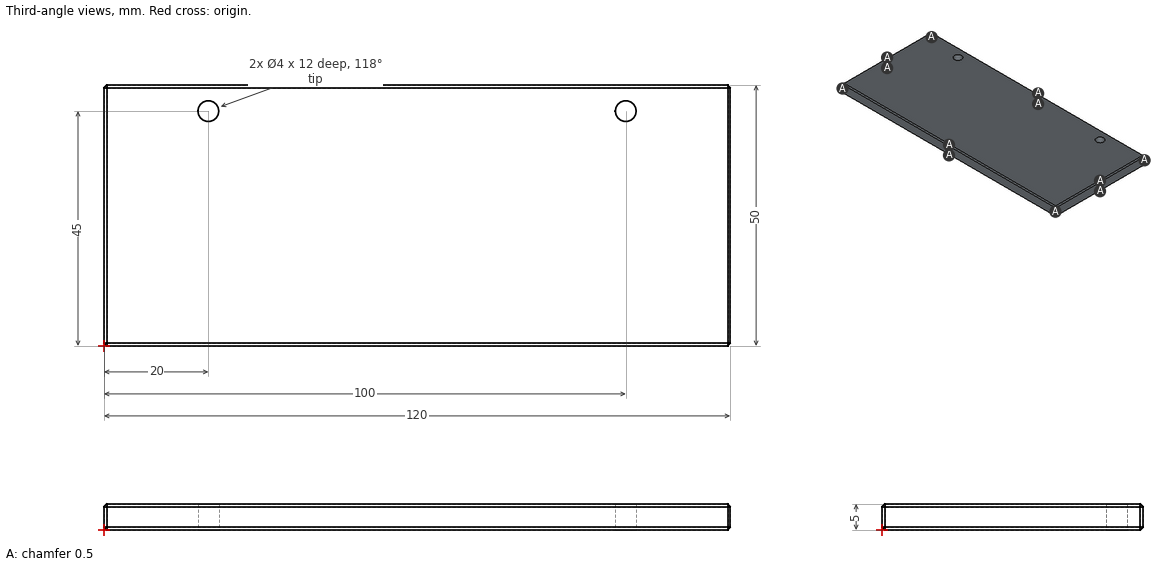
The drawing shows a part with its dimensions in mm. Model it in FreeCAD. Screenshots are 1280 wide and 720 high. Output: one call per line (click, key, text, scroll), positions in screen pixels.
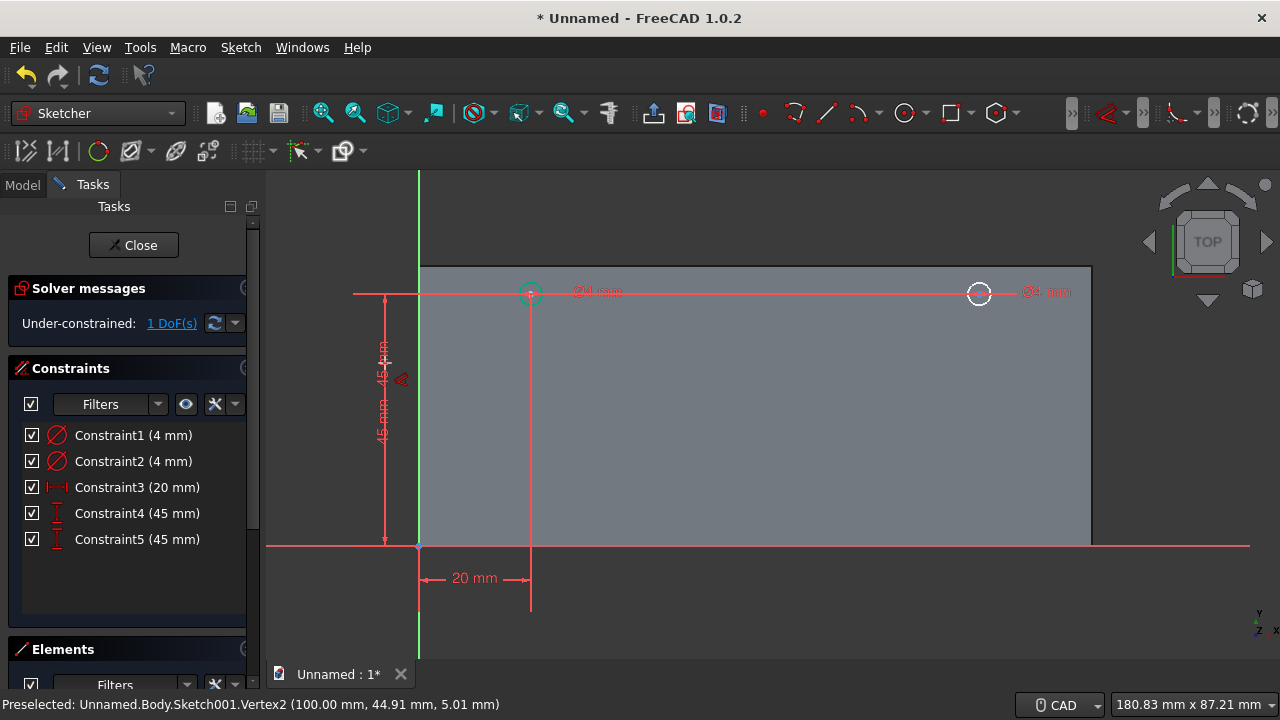
click(979, 294)
click(699, 580)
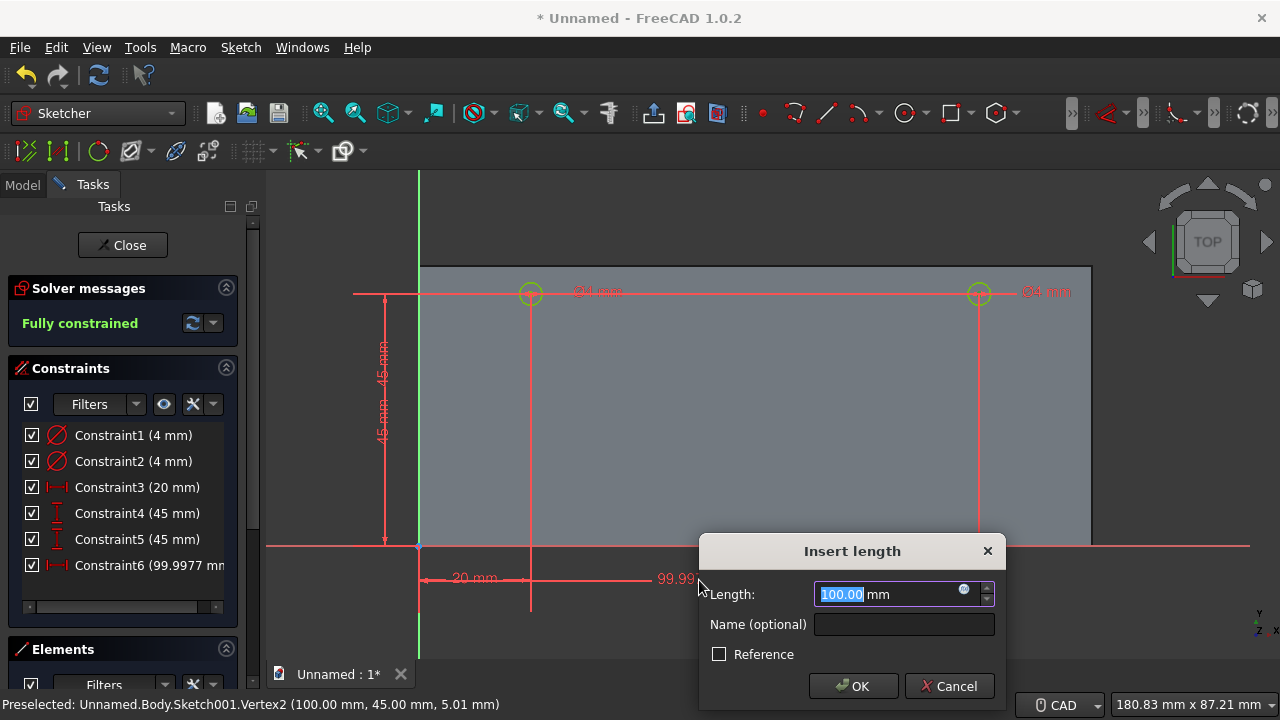
text(100)
key(Return)
key(Escape)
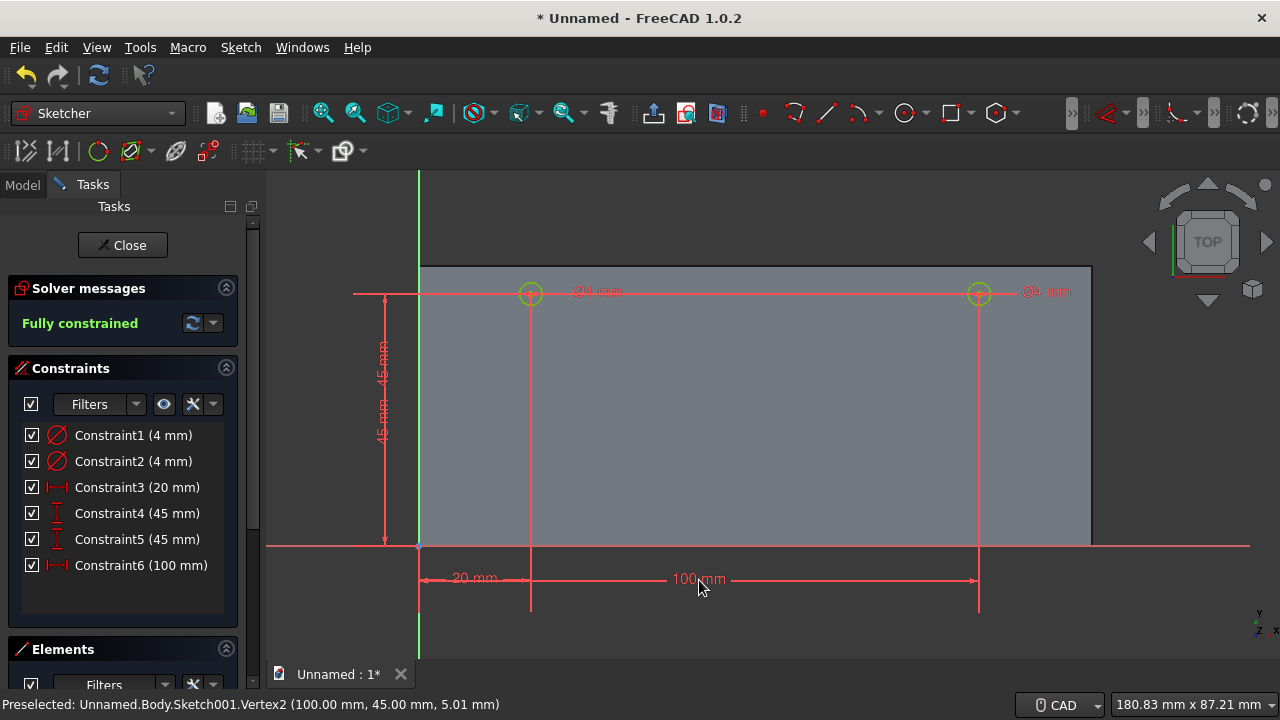
click(123, 245)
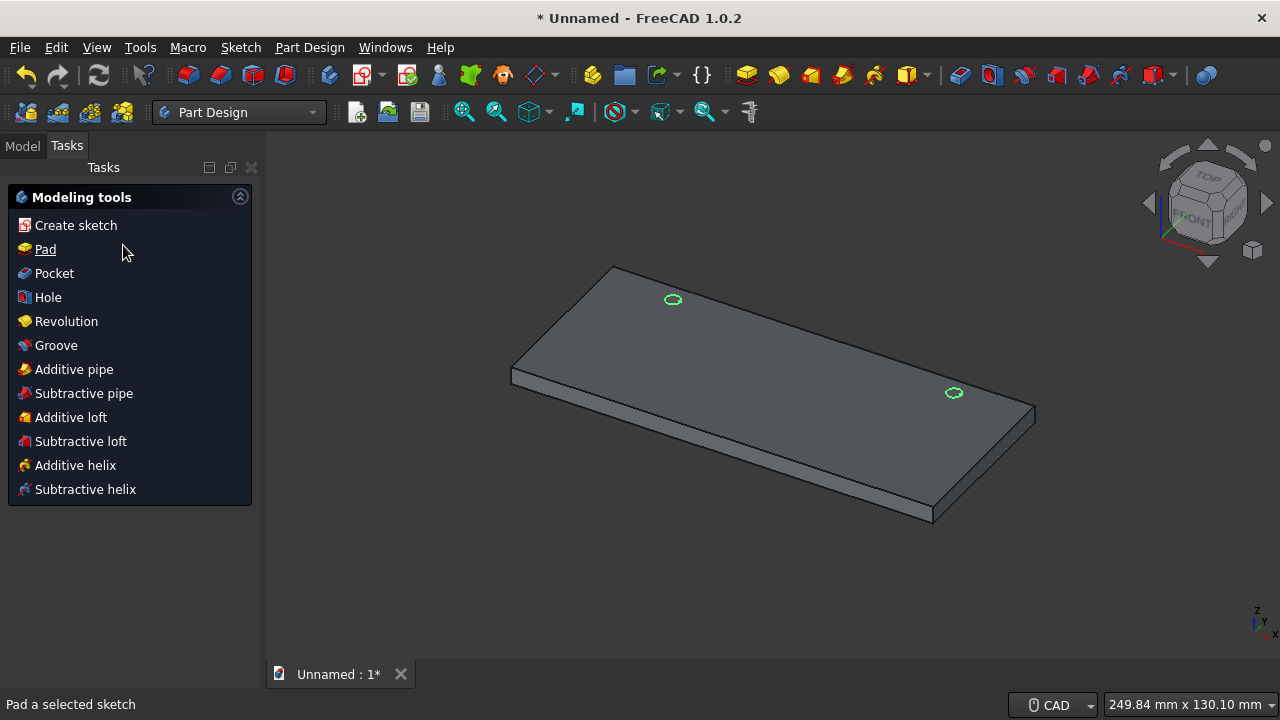
click(994, 76)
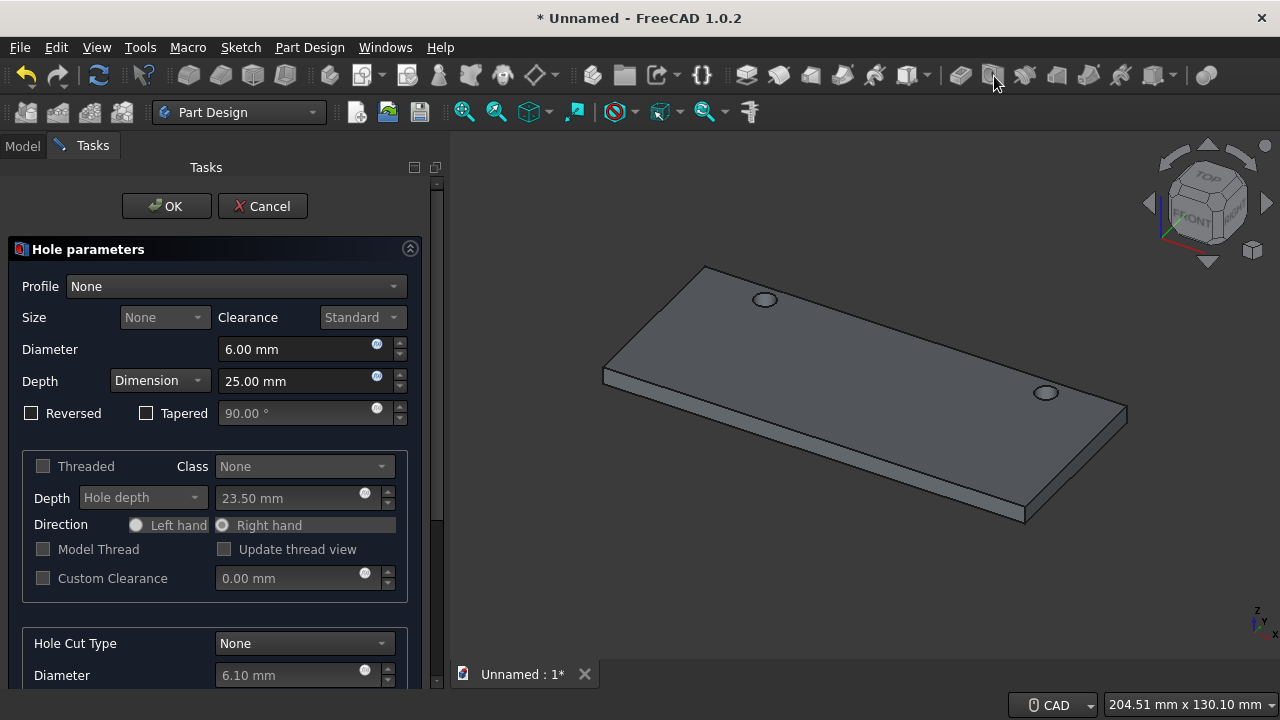
triple_click(305, 349)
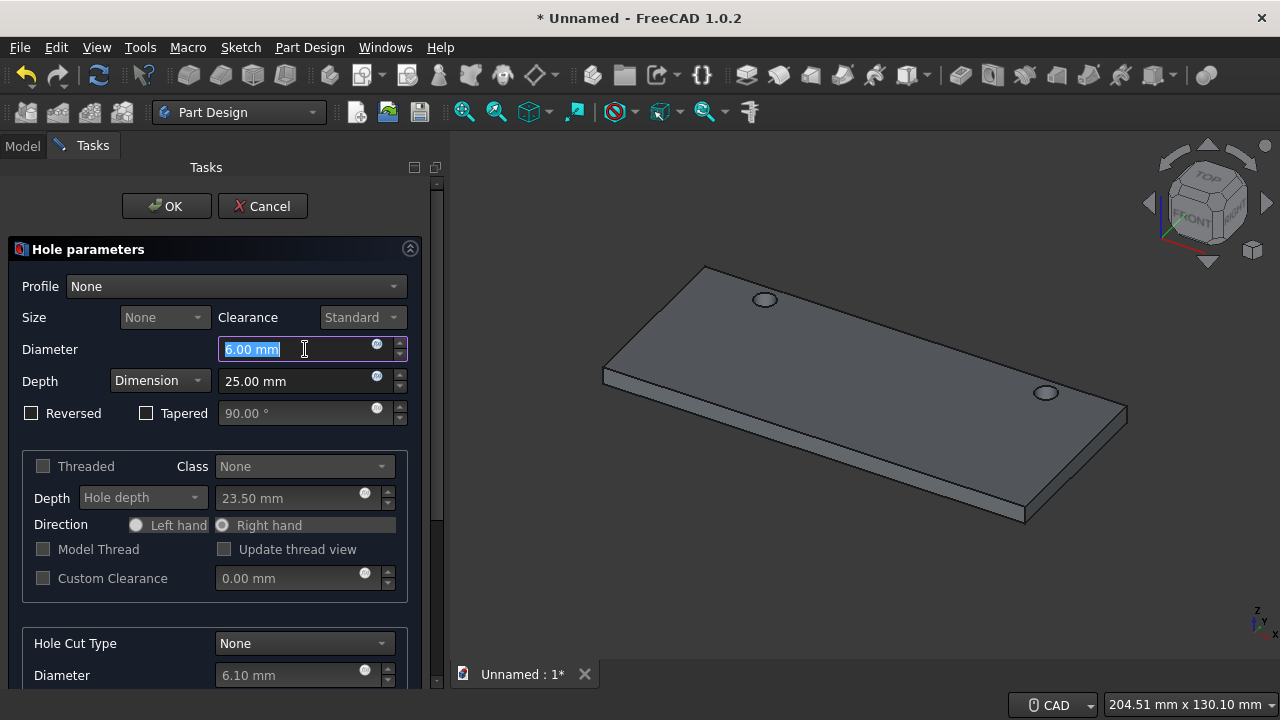
text(4)
key(Tab)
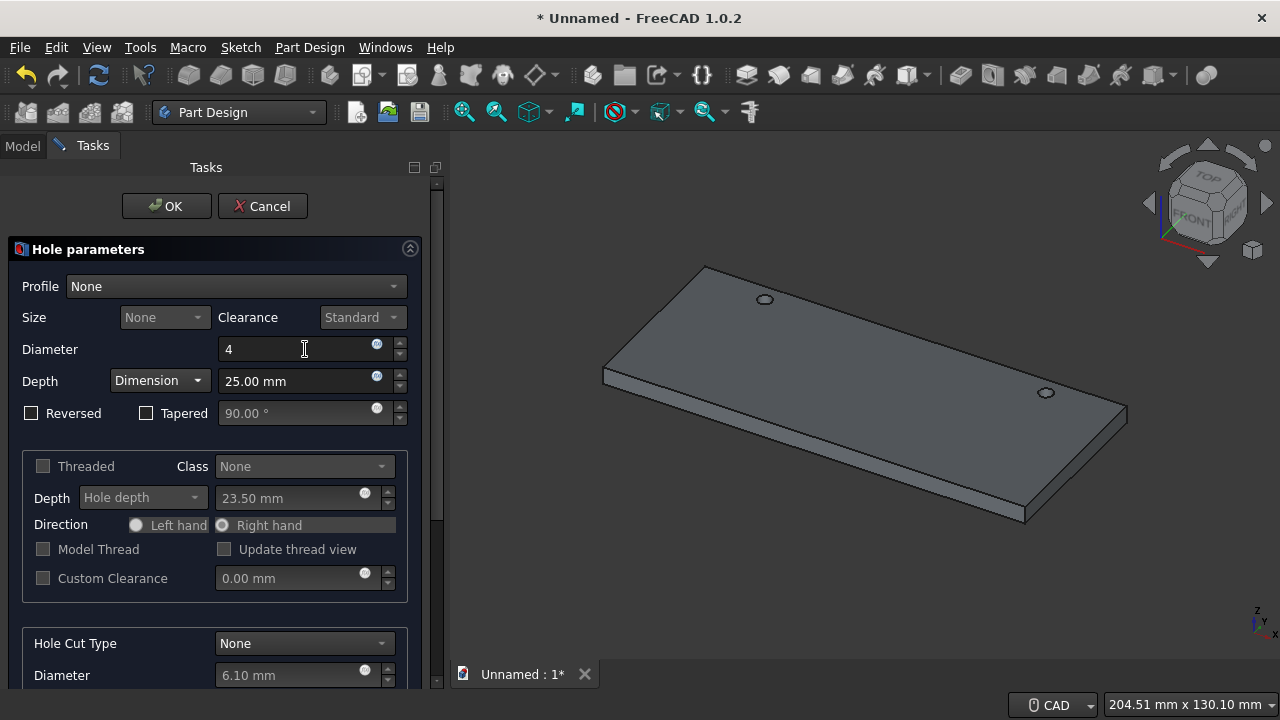
triple_click(305, 381)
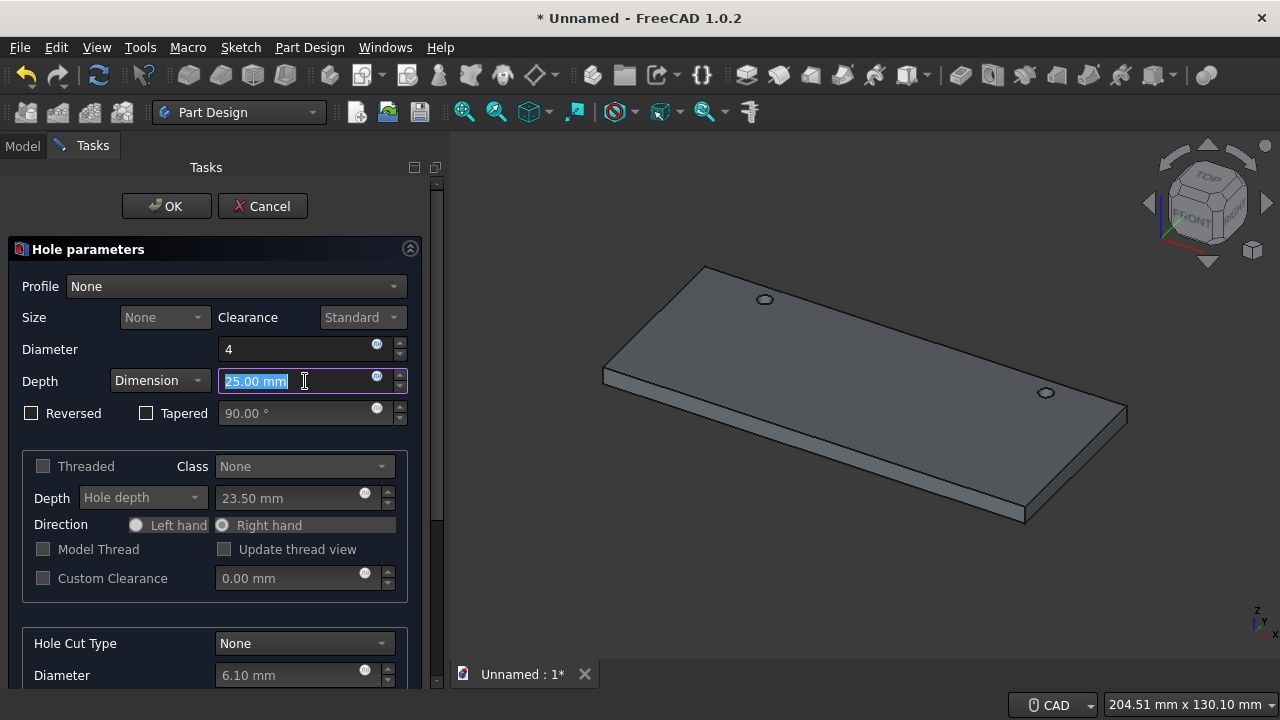
text(12)
key(Tab)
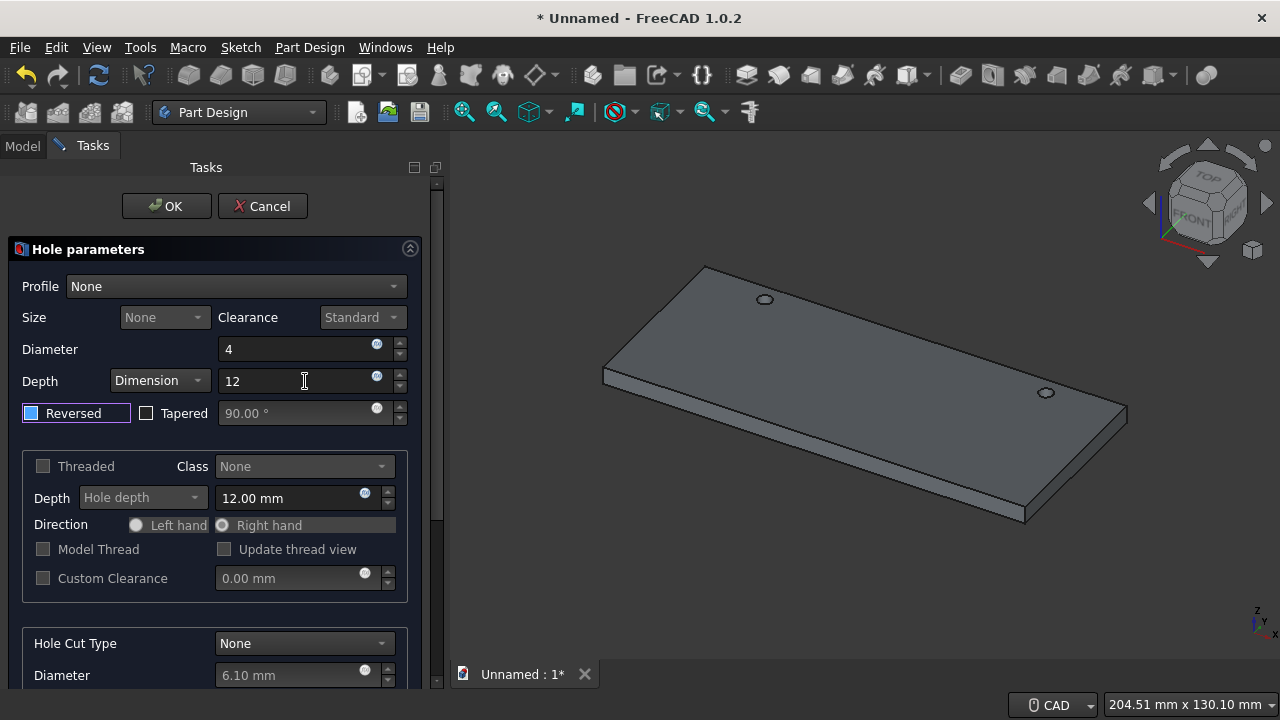
click(167, 206)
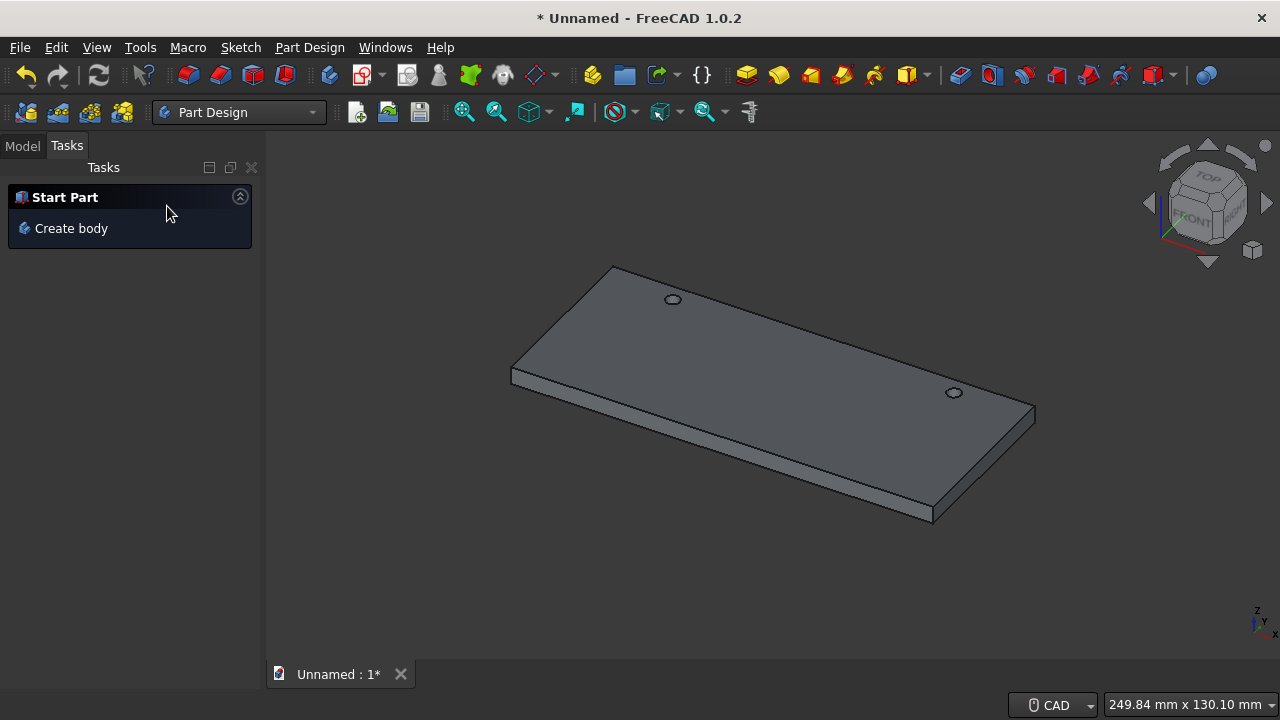
click(984, 456)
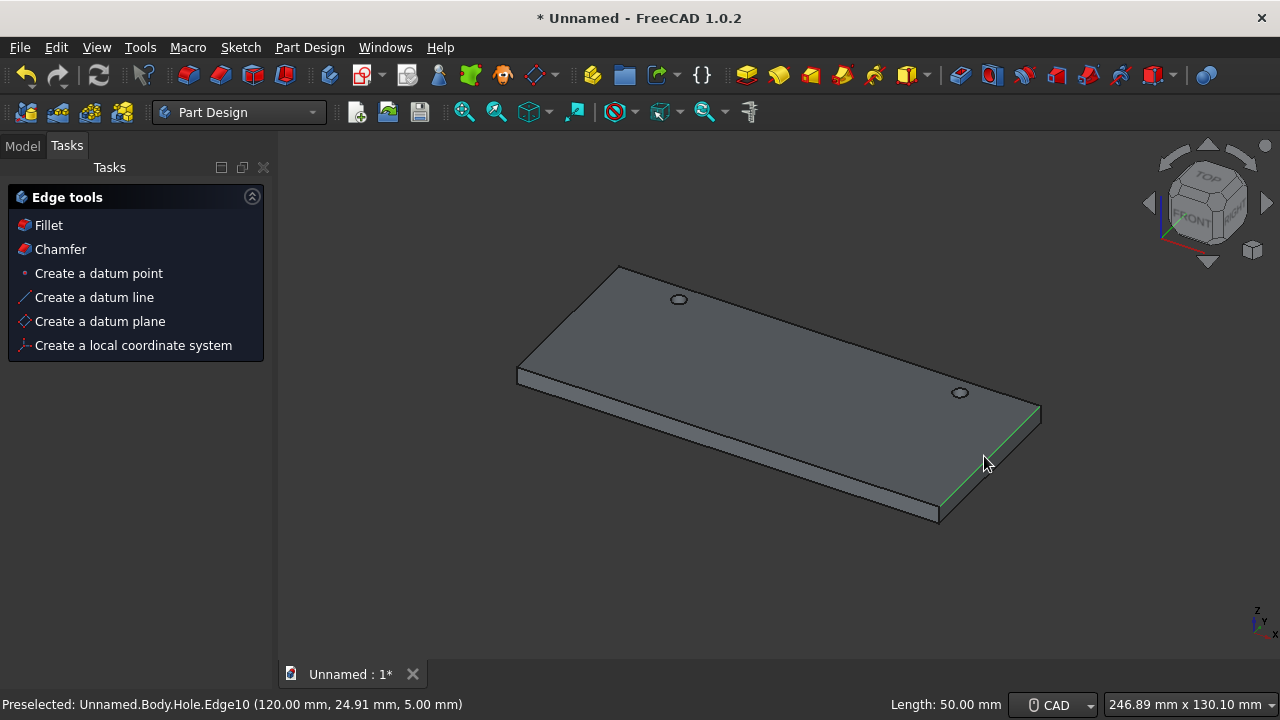
key(0)